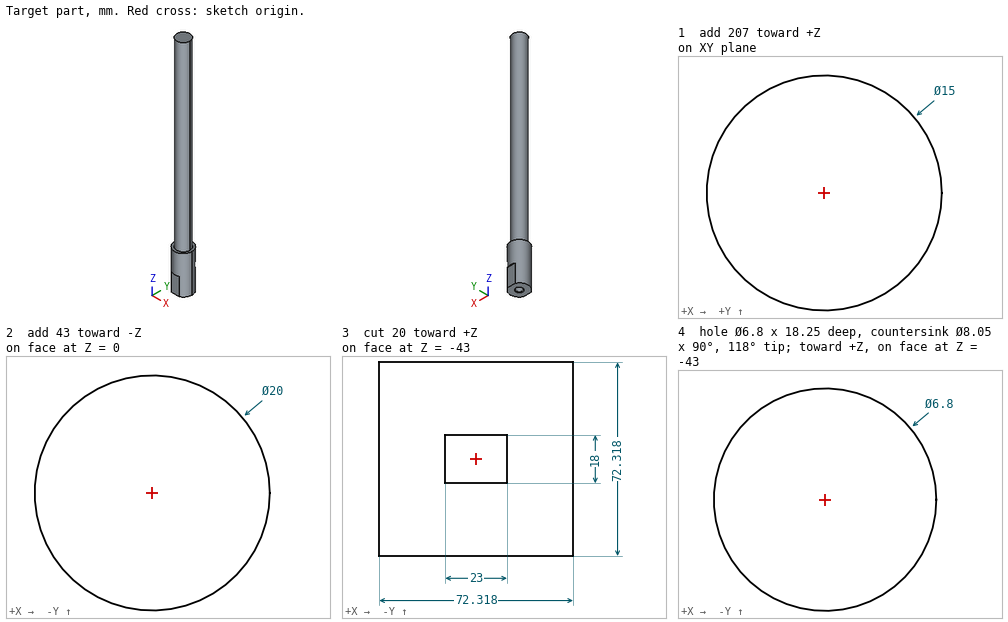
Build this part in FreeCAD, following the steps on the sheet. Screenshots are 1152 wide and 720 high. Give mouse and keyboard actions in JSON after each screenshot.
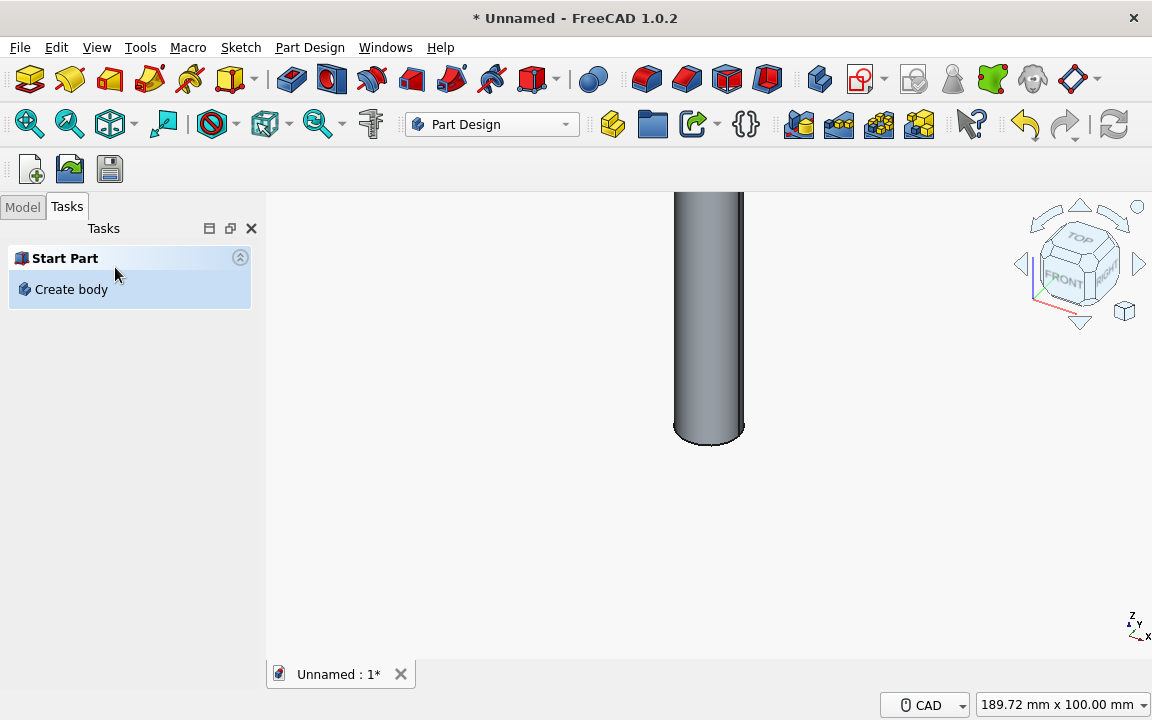
{"action": "key", "text": "v f"}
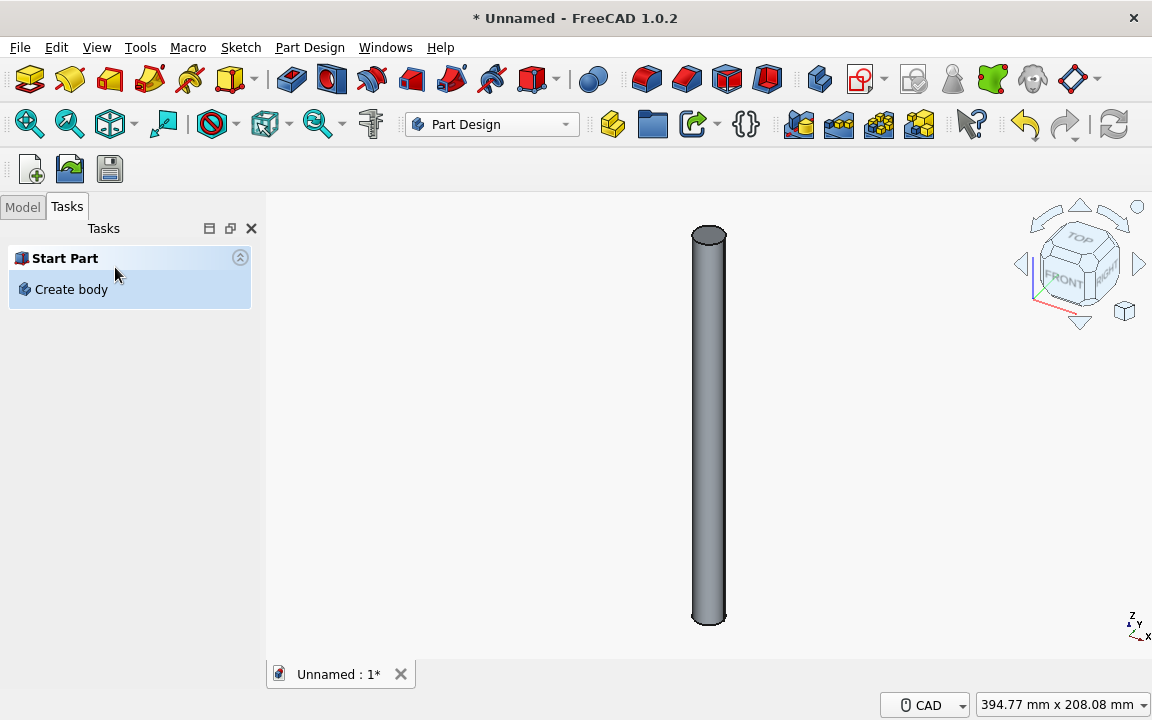
{"action": "key", "text": "5"}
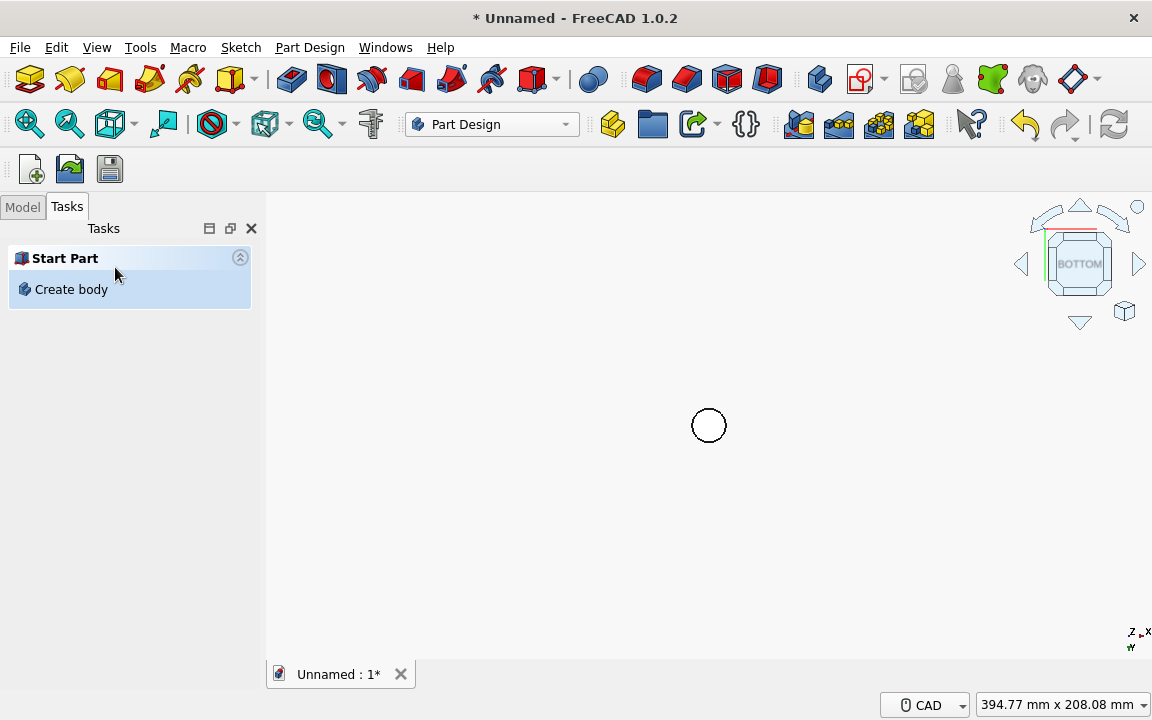
{"action": "key", "text": "v f"}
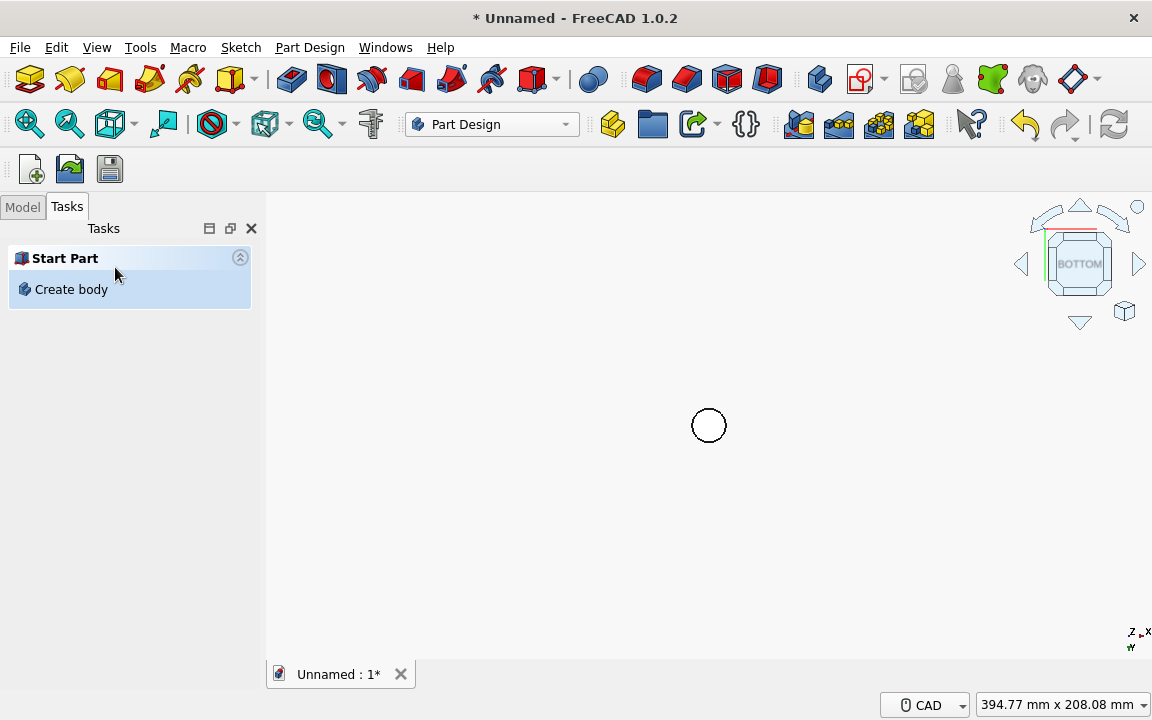
{"action": "left_click", "coordinate": [709, 424]}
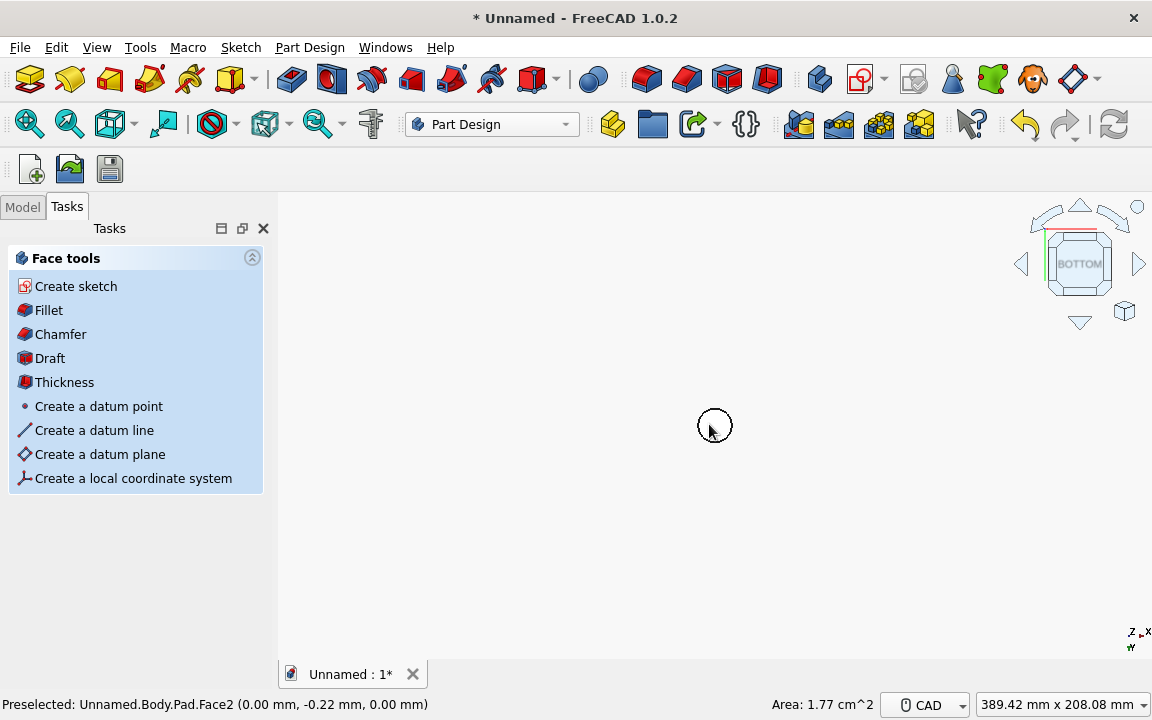
{"action": "left_click", "coordinate": [860, 80]}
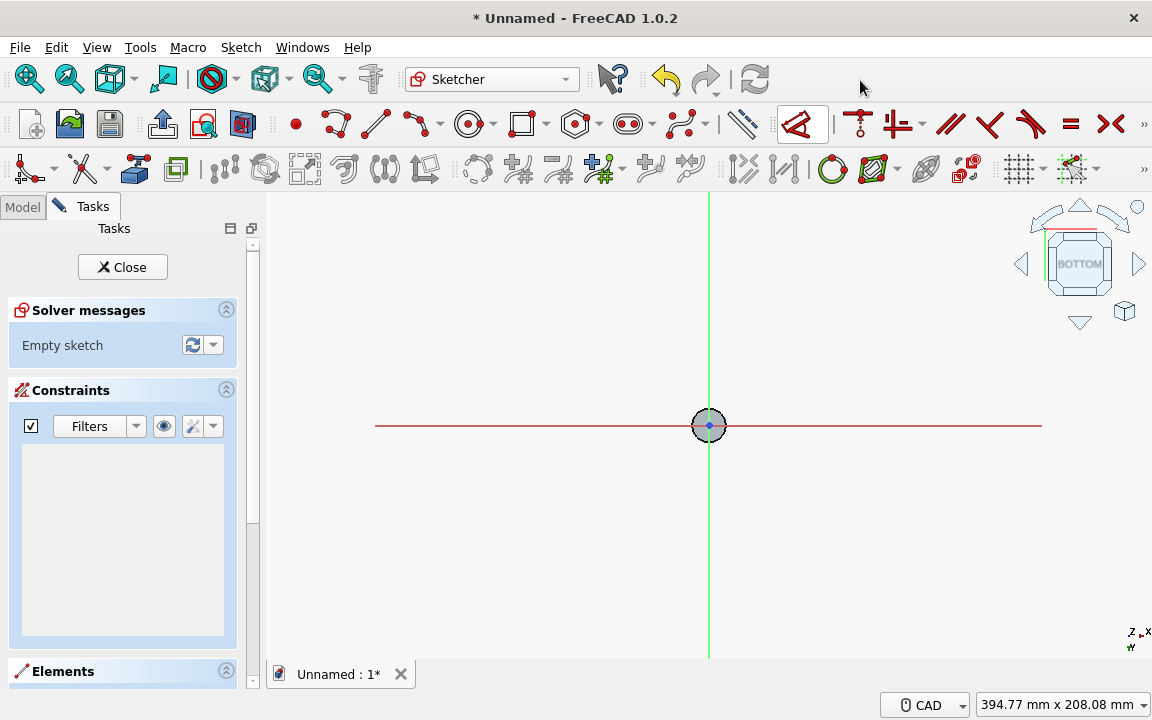
{"action": "scroll", "coordinate": [723, 426], "scroll_direction": "up", "scroll_amount": 9}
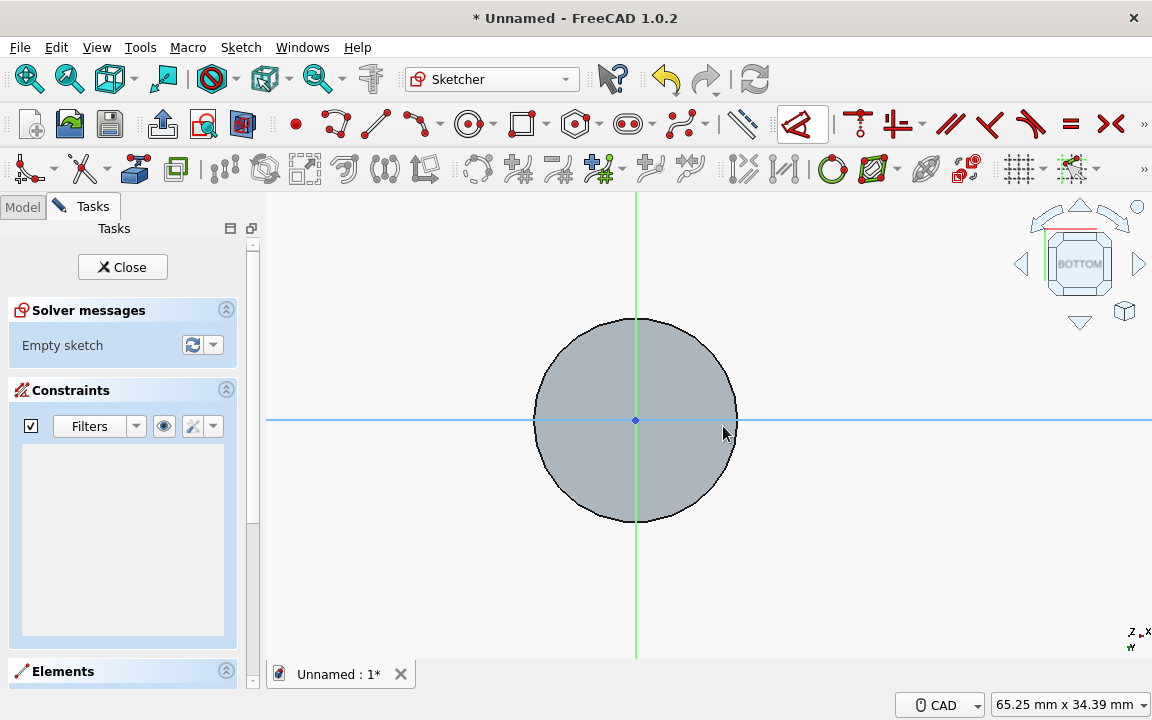
{"action": "key", "text": "g c"}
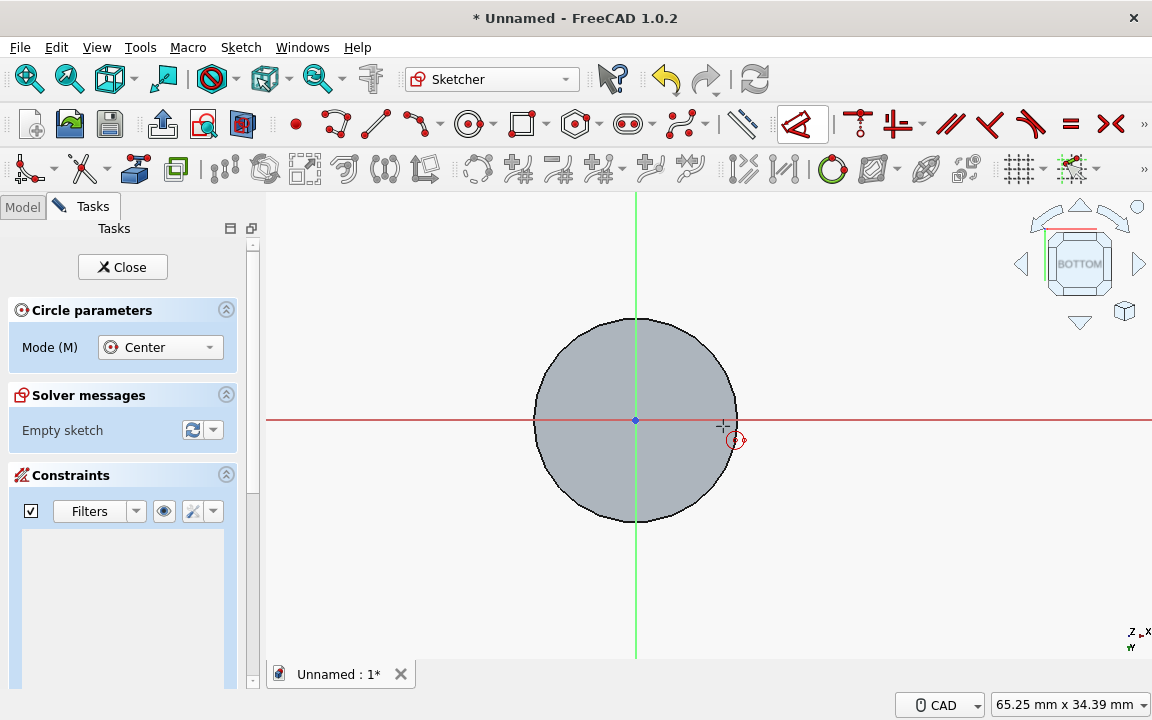
{"action": "left_click", "coordinate": [636, 420]}
{"action": "mouse_move", "coordinate": [732, 324]}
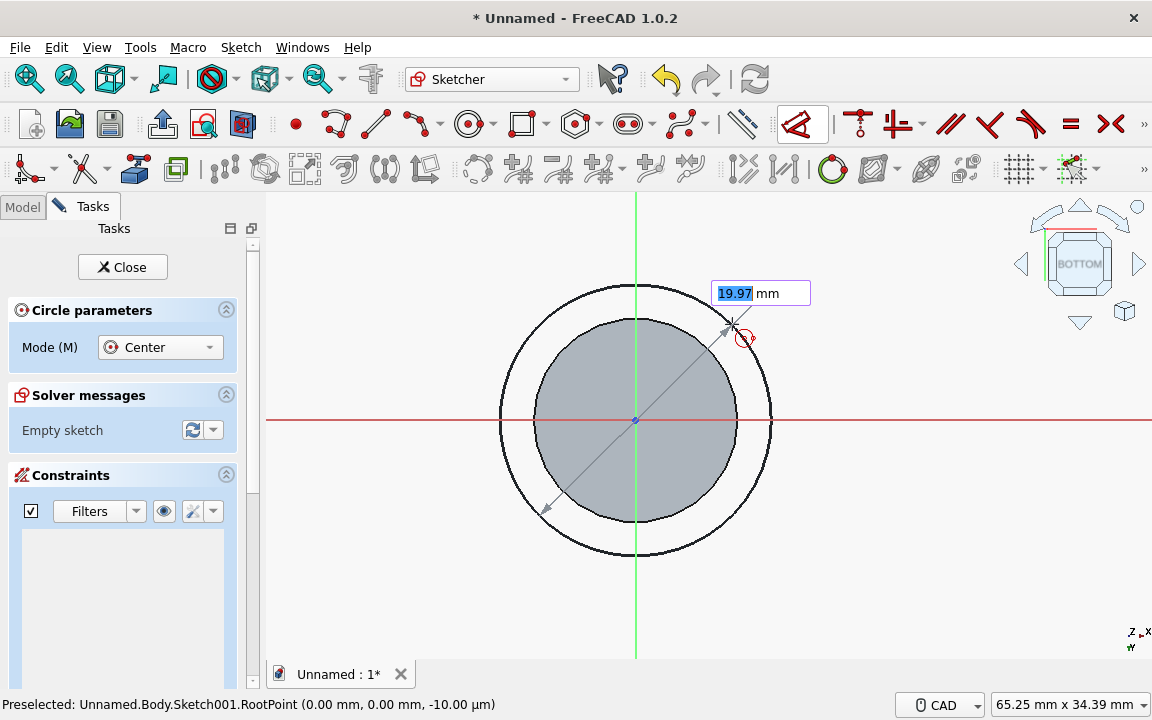
{"action": "type", "text": "20"}
{"action": "key", "text": "Return"}
{"action": "key", "text": "Escape"}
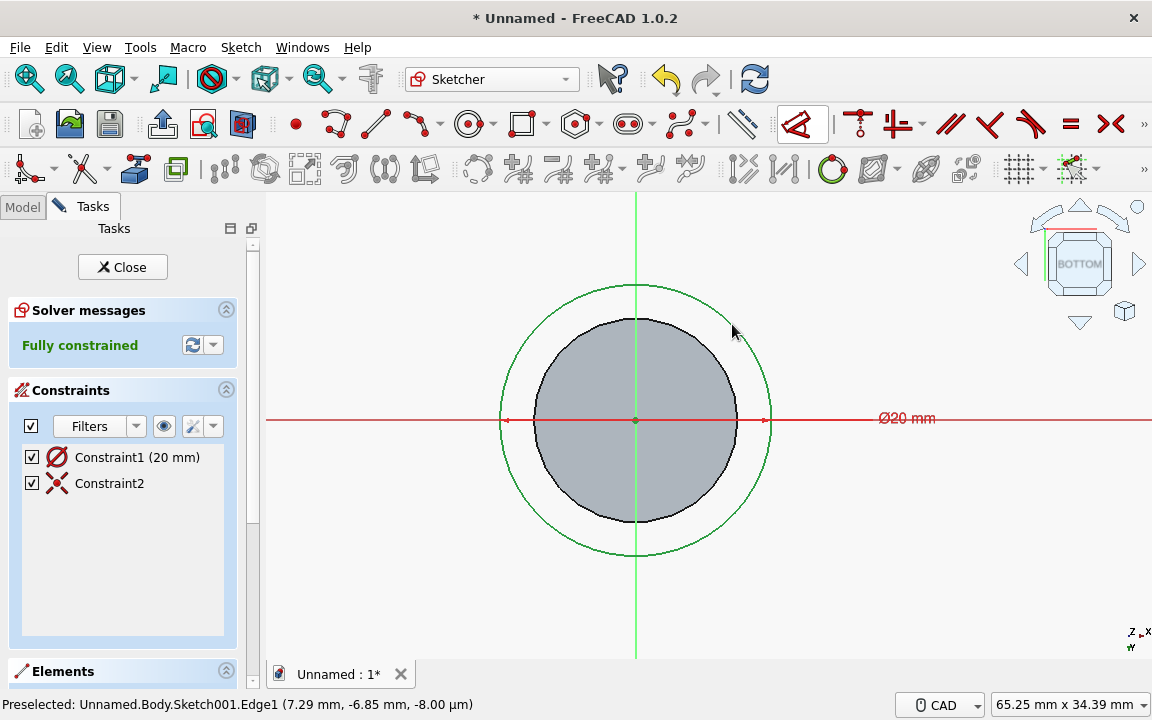
{"action": "left_click", "coordinate": [123, 267]}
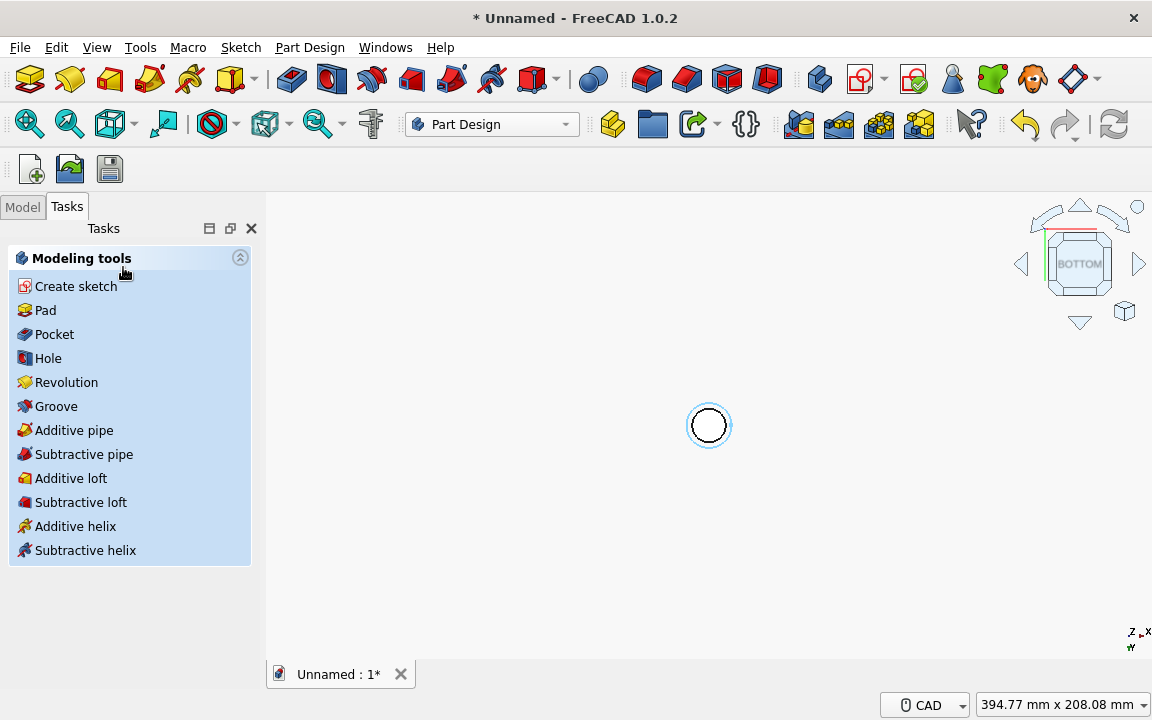
{"action": "left_click", "coordinate": [30, 80]}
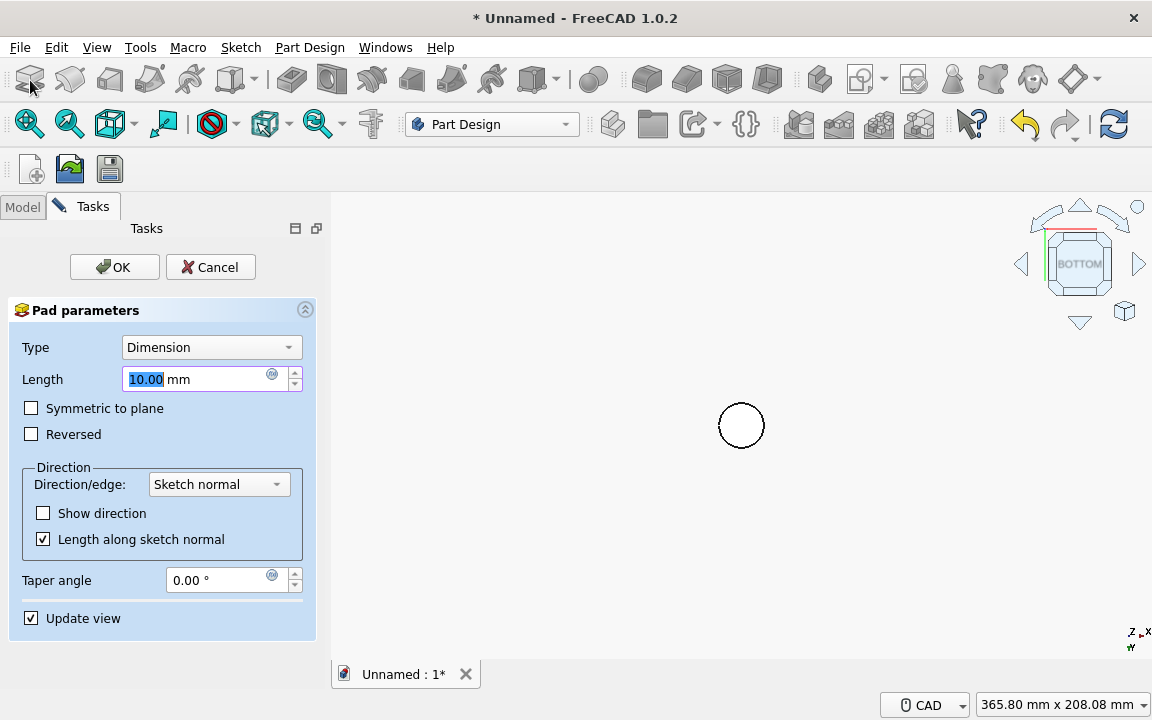
{"action": "type", "text": "43"}
{"action": "key", "text": "Tab"}